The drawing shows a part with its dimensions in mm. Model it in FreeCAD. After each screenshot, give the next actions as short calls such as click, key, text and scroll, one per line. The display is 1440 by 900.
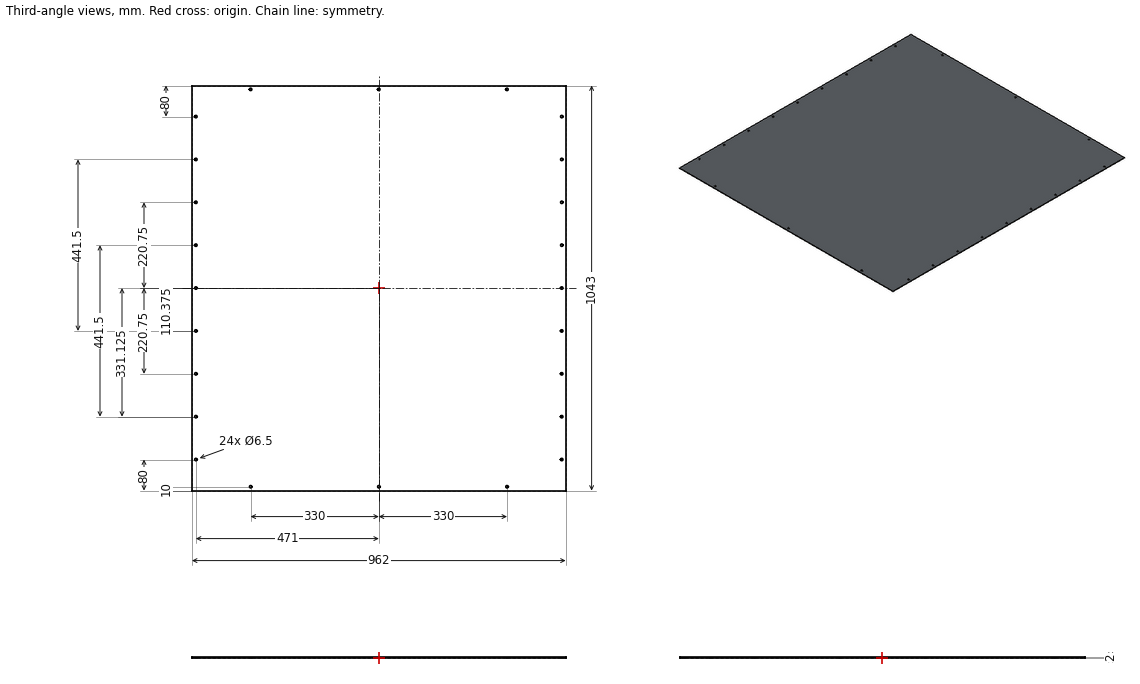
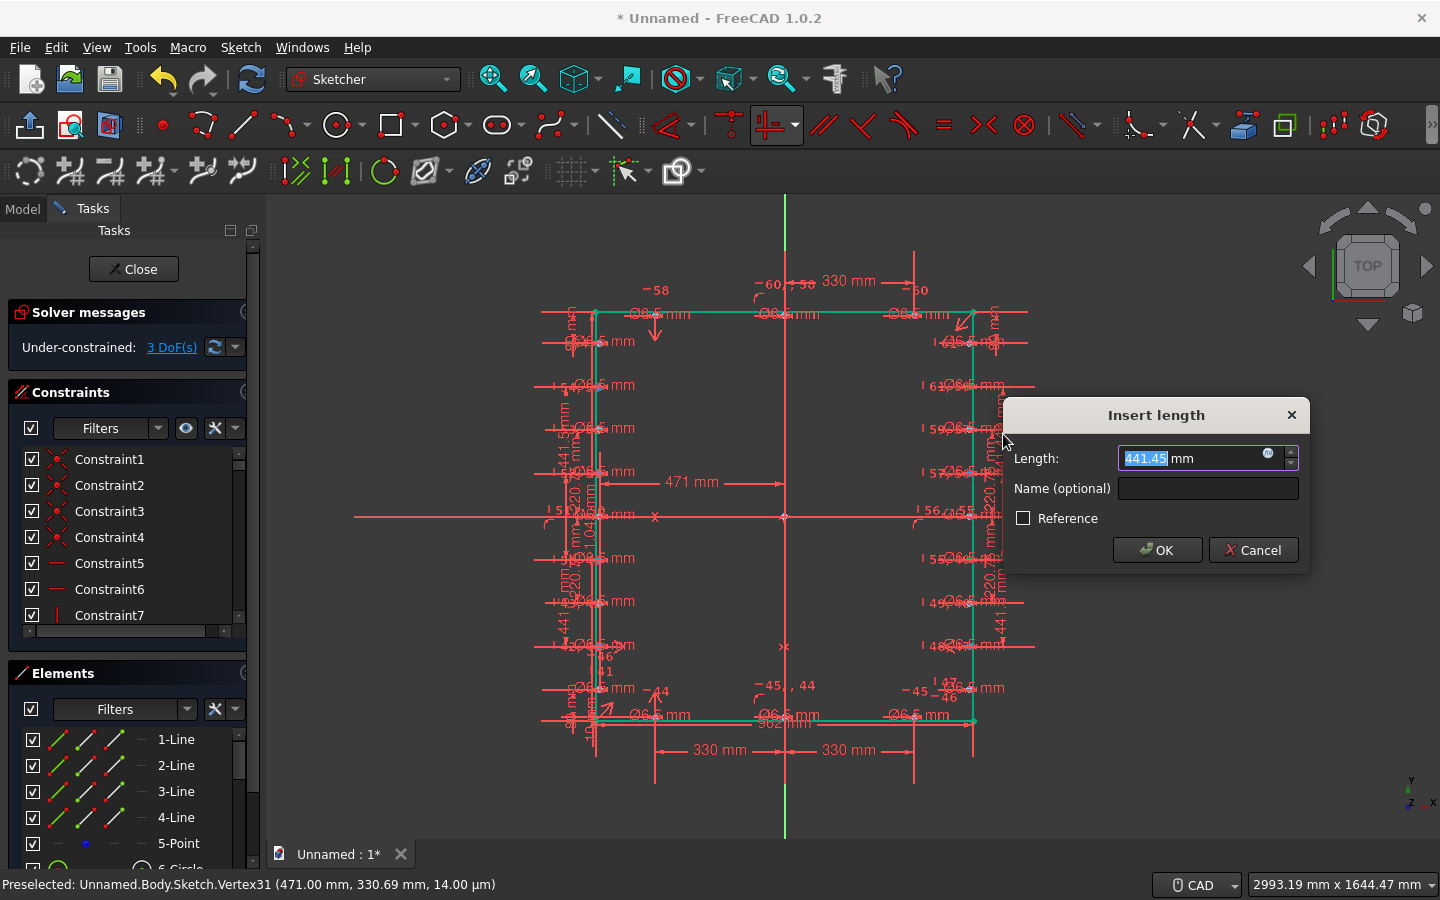
text(441.5)
key(Return)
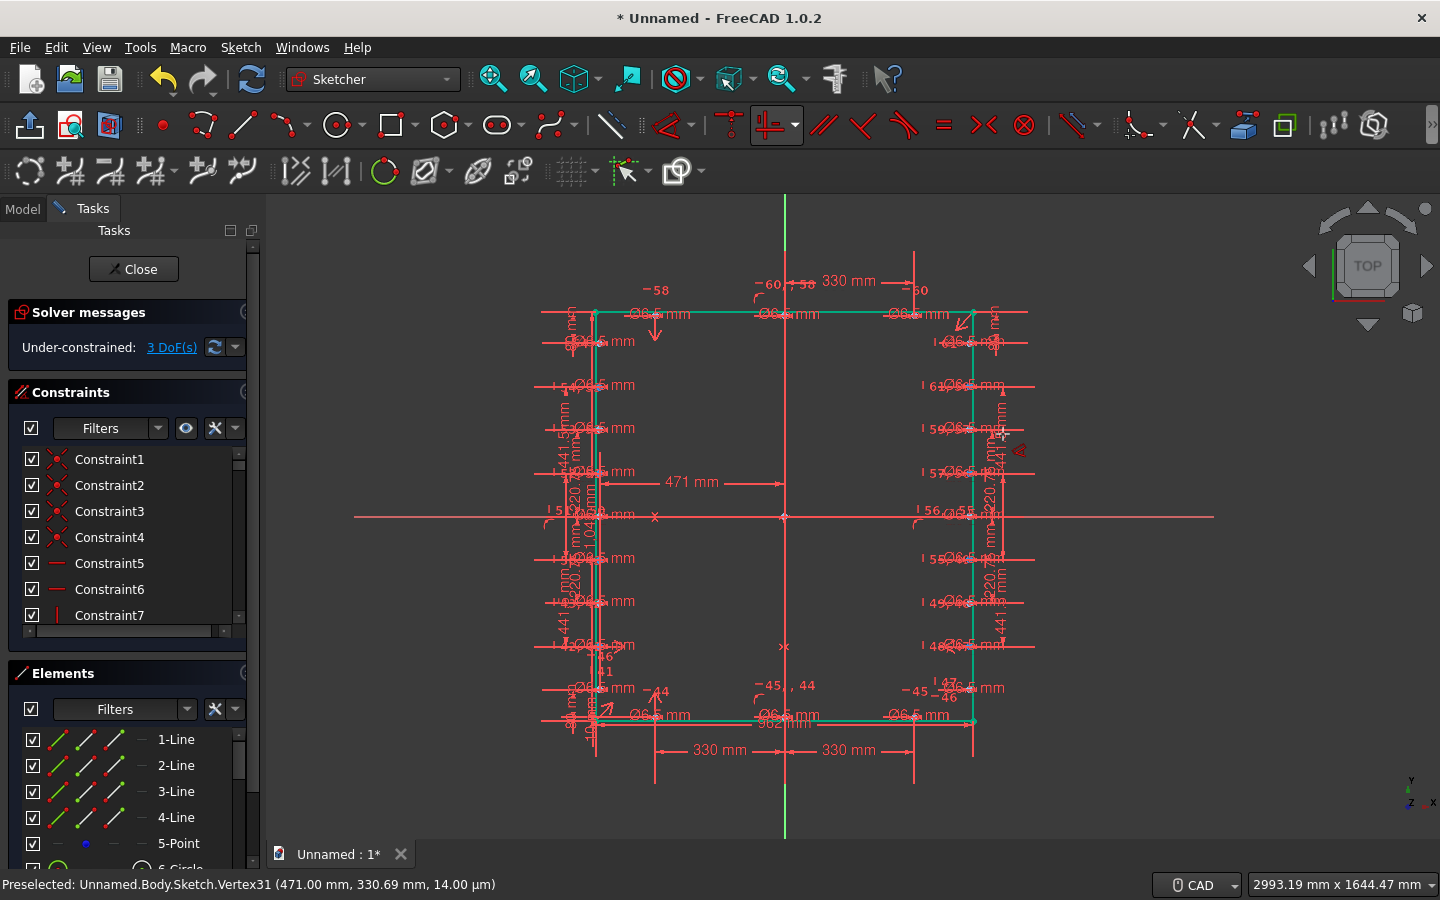
click(600, 647)
click(566, 536)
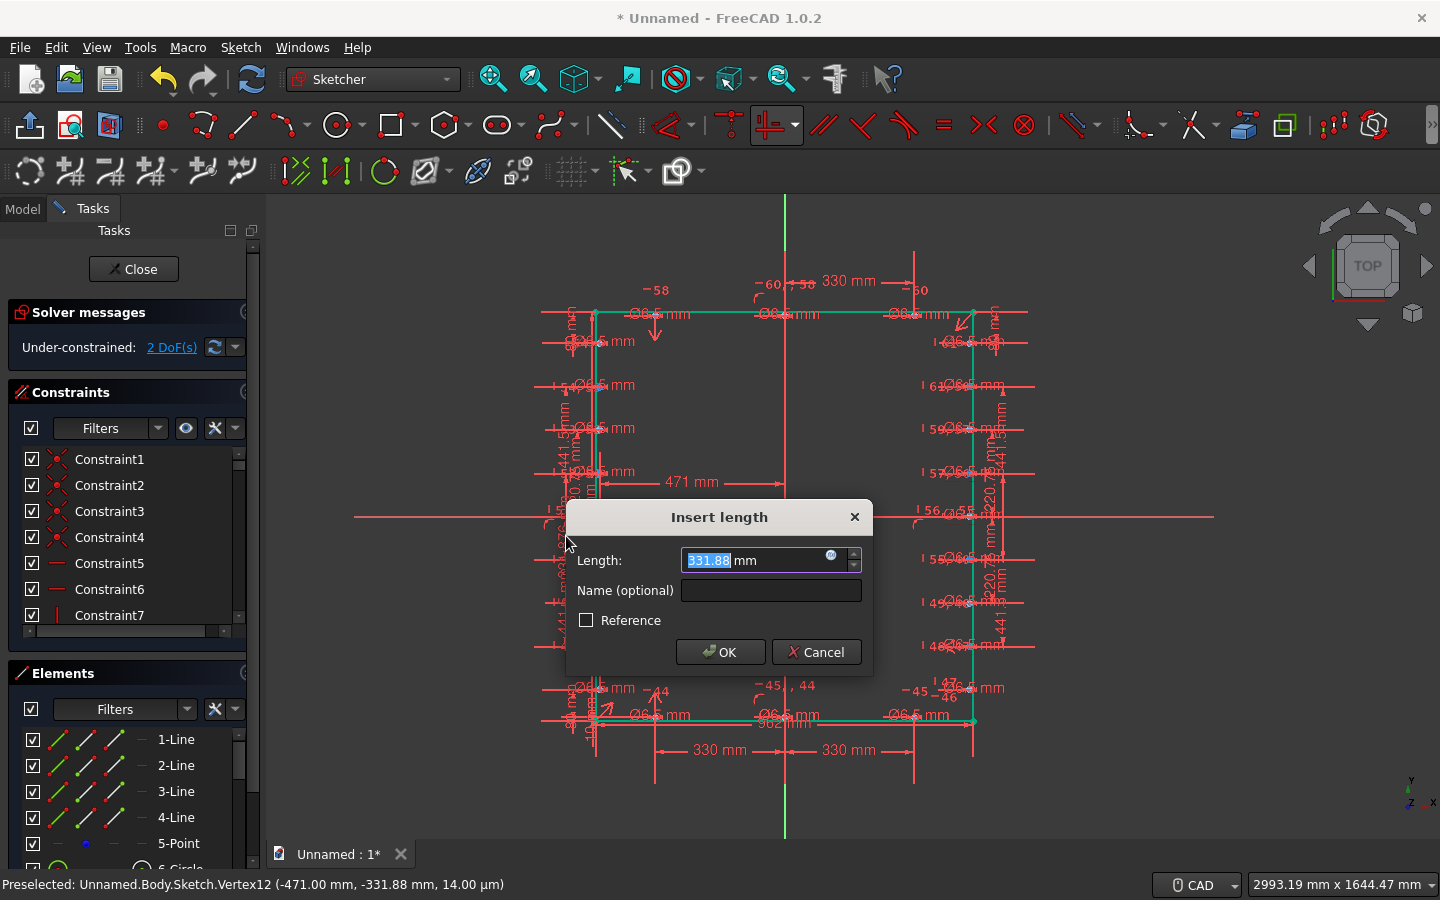
text(331.125)
key(Return)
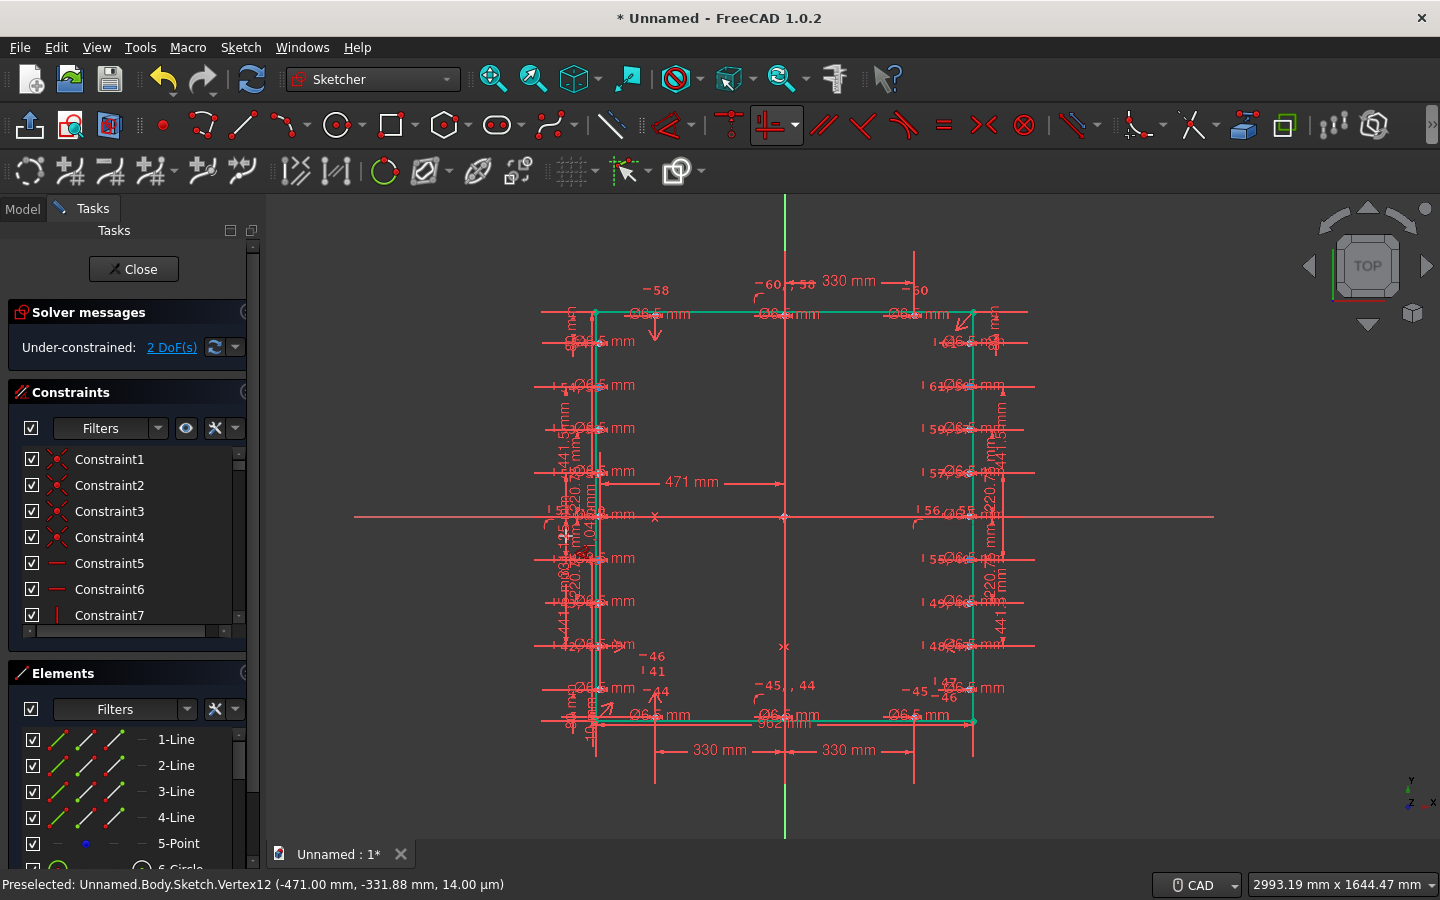
click(600, 560)
click(819, 538)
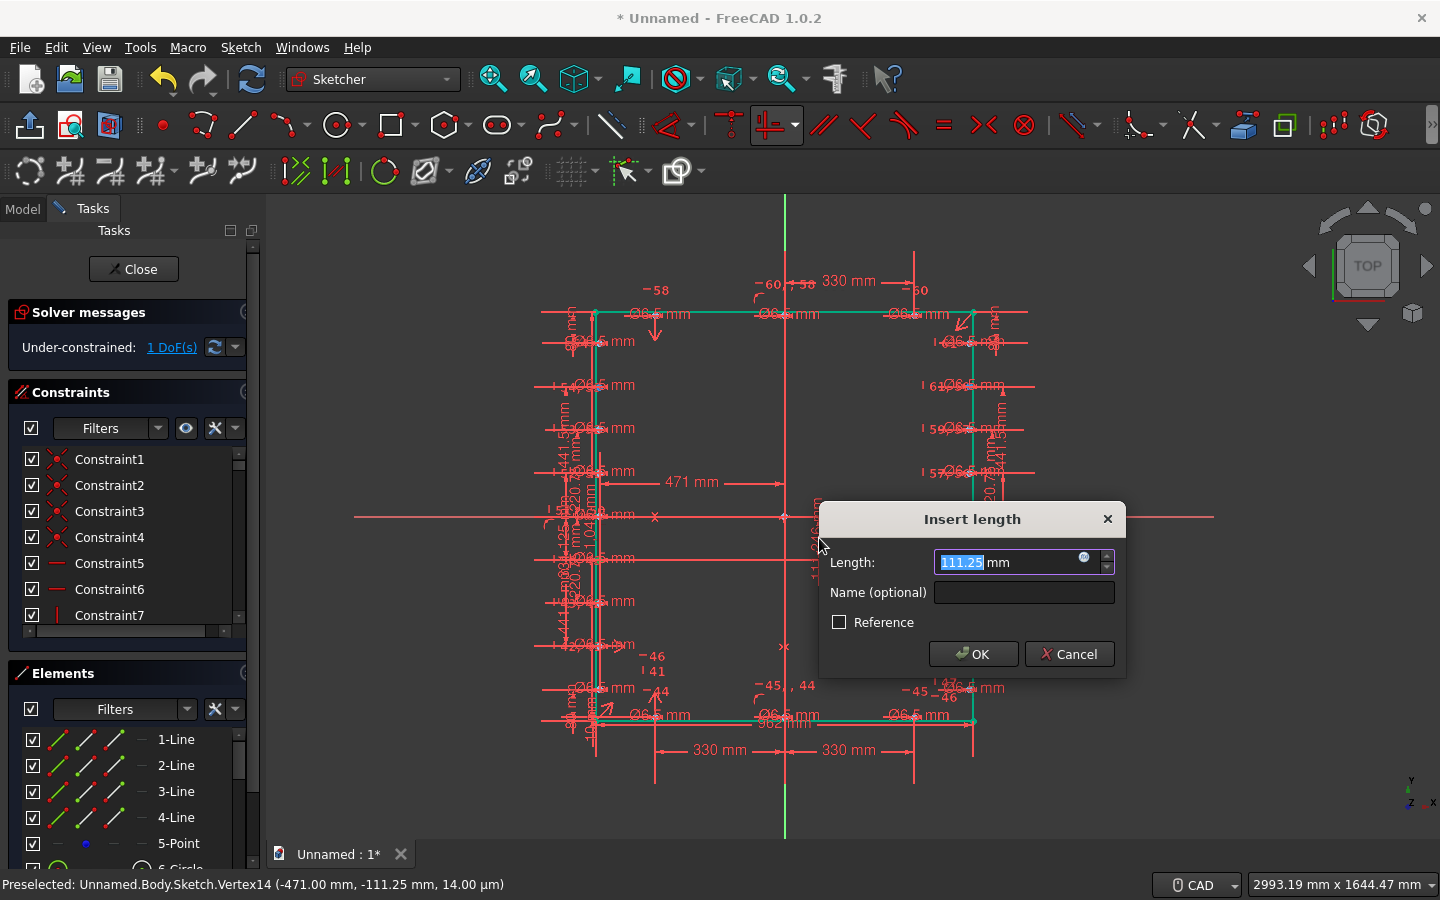
text(110.375)
key(Return)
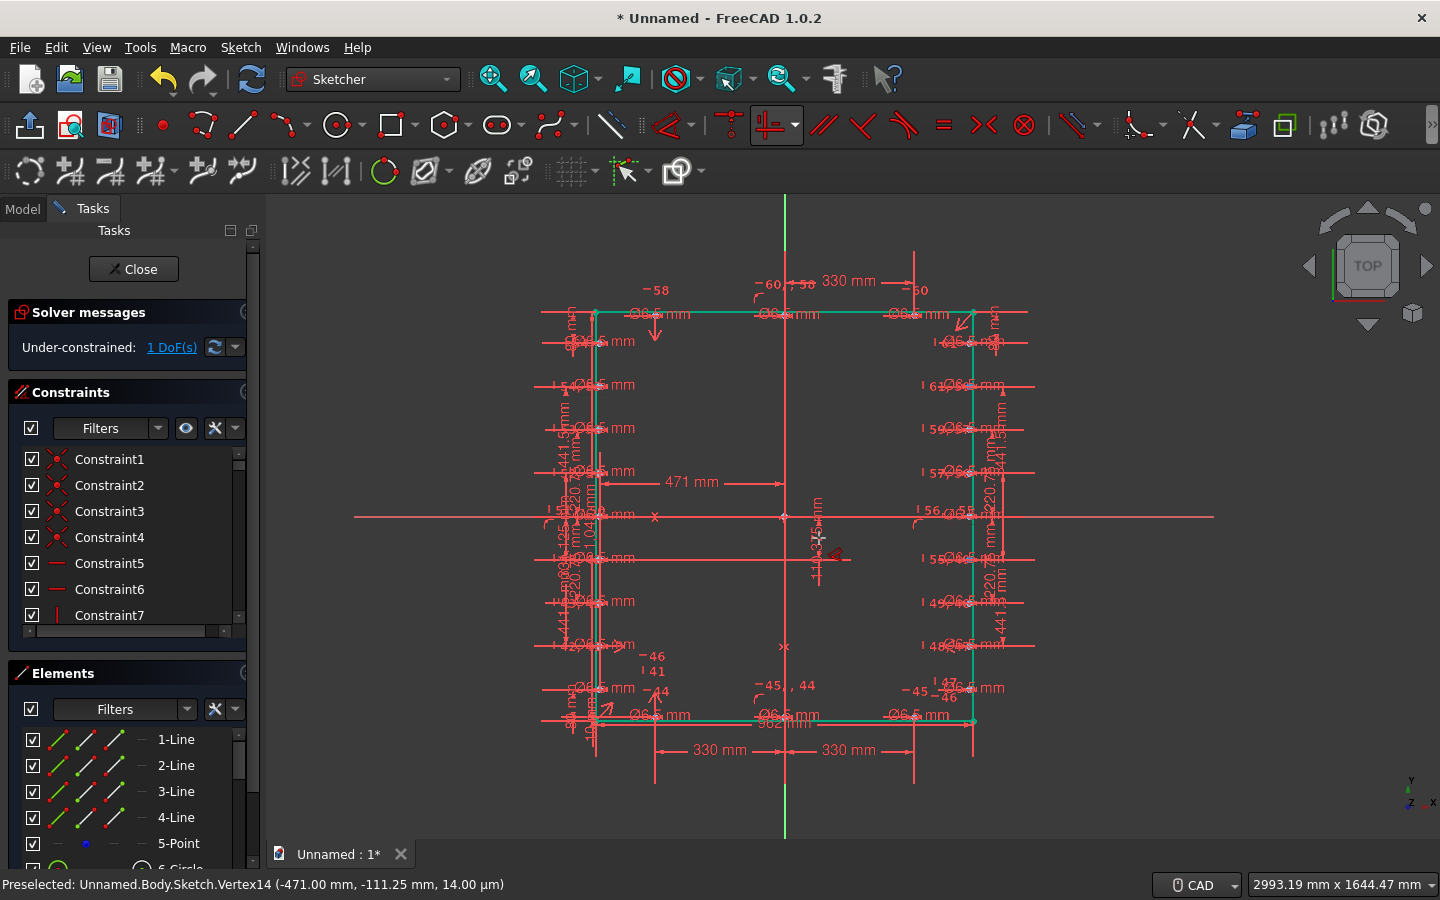
click(969, 560)
click(1003, 538)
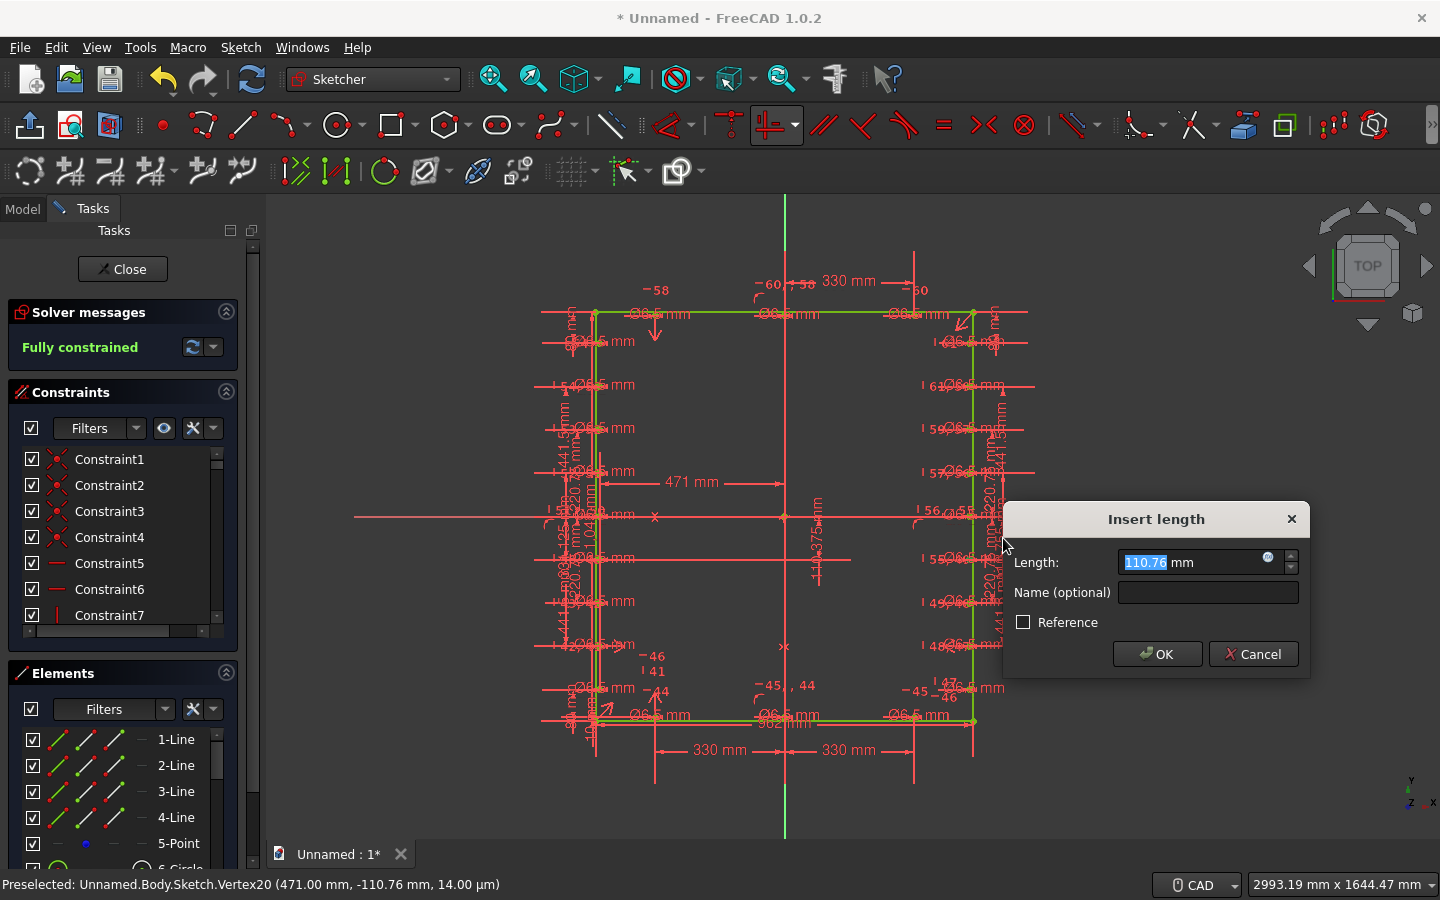
text(110.375)
key(Return)
key(Escape)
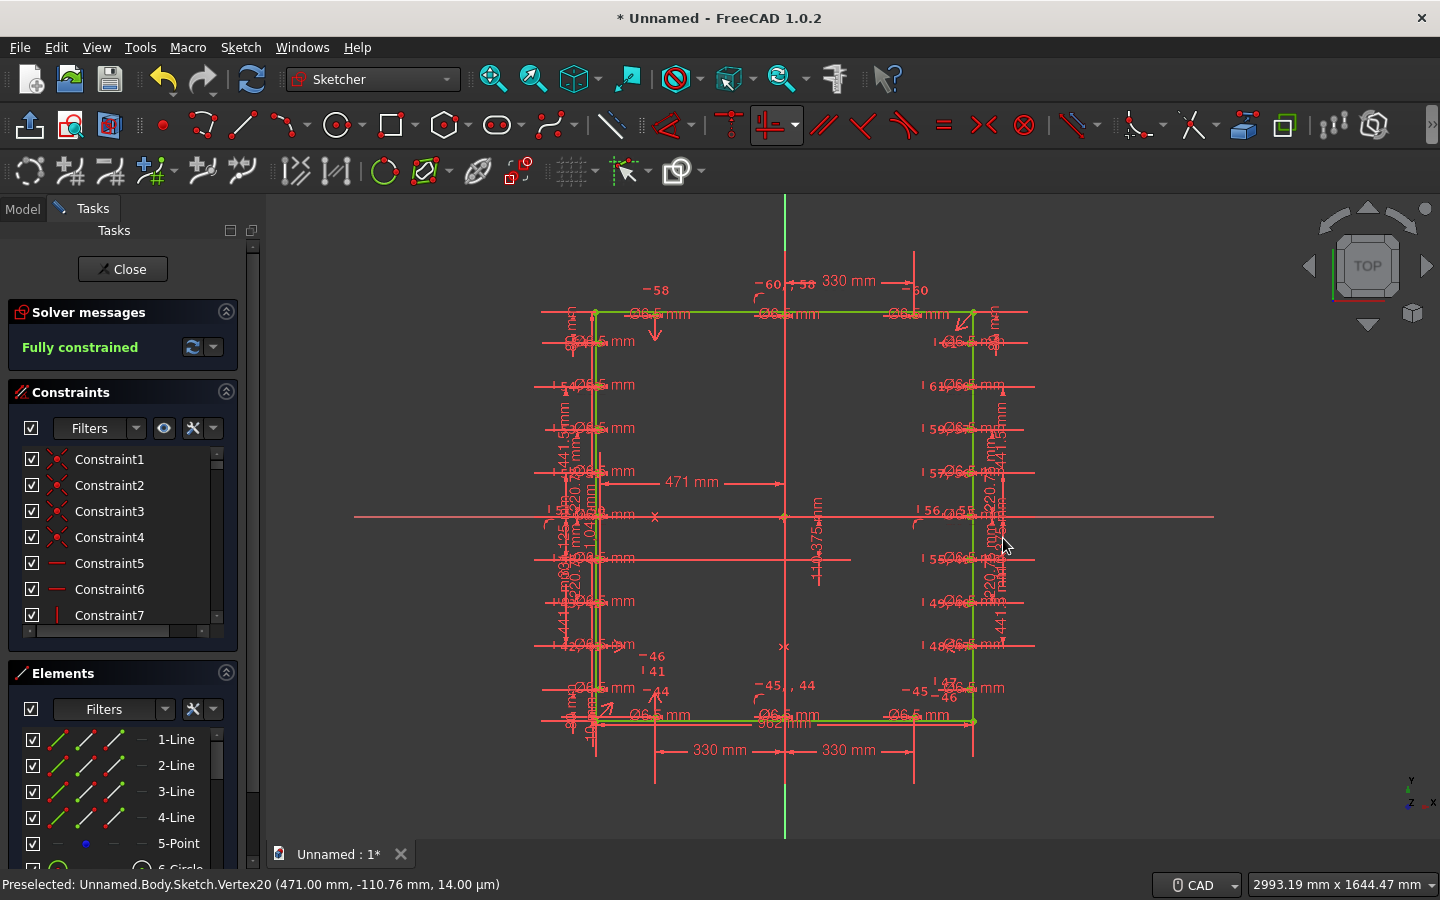
click(123, 269)